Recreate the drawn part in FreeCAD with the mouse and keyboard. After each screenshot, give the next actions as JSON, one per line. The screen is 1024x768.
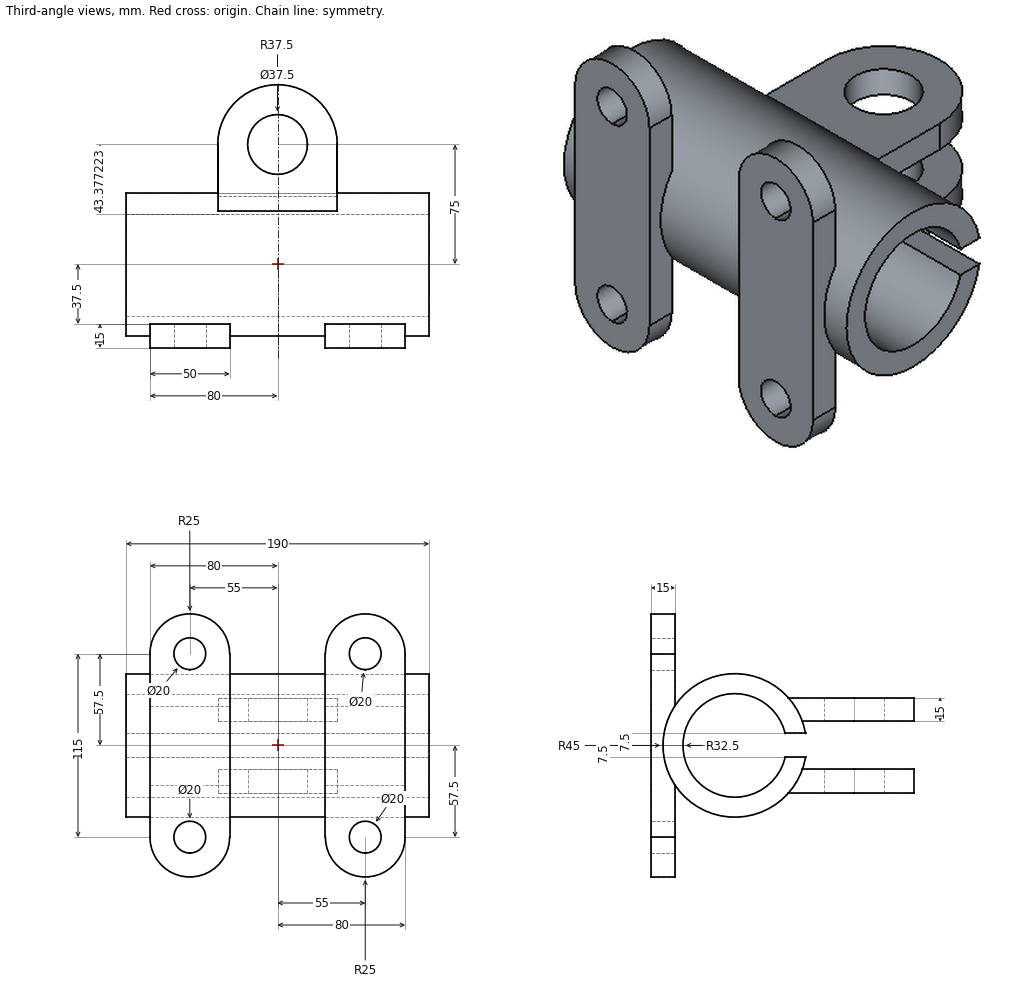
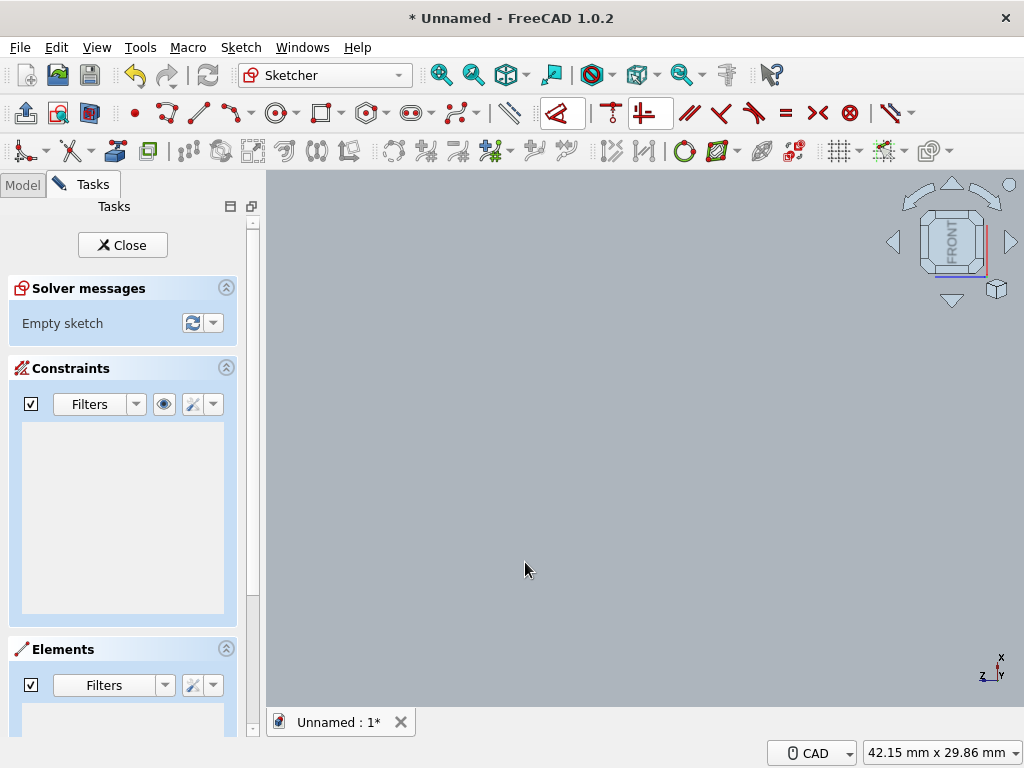
{"action": "left_click", "coordinate": [276, 114]}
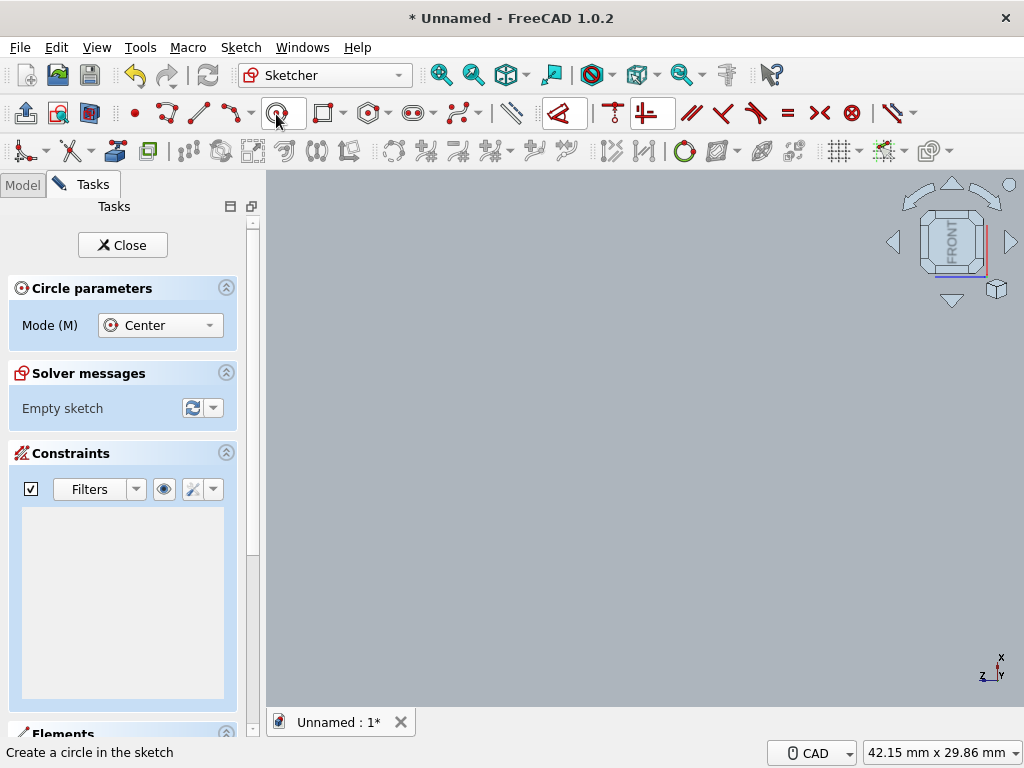
{"action": "left_click", "coordinate": [571, 431]}
{"action": "left_click", "coordinate": [698, 304]}
{"action": "key", "text": "Escape"}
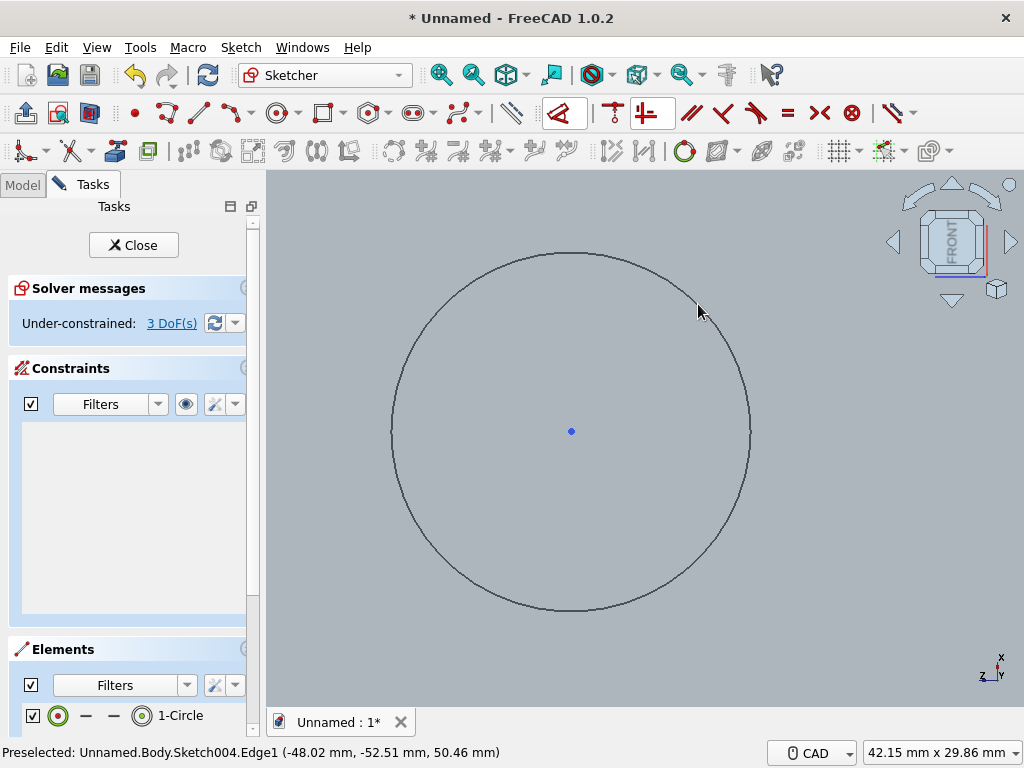
{"action": "left_click", "coordinate": [698, 305]}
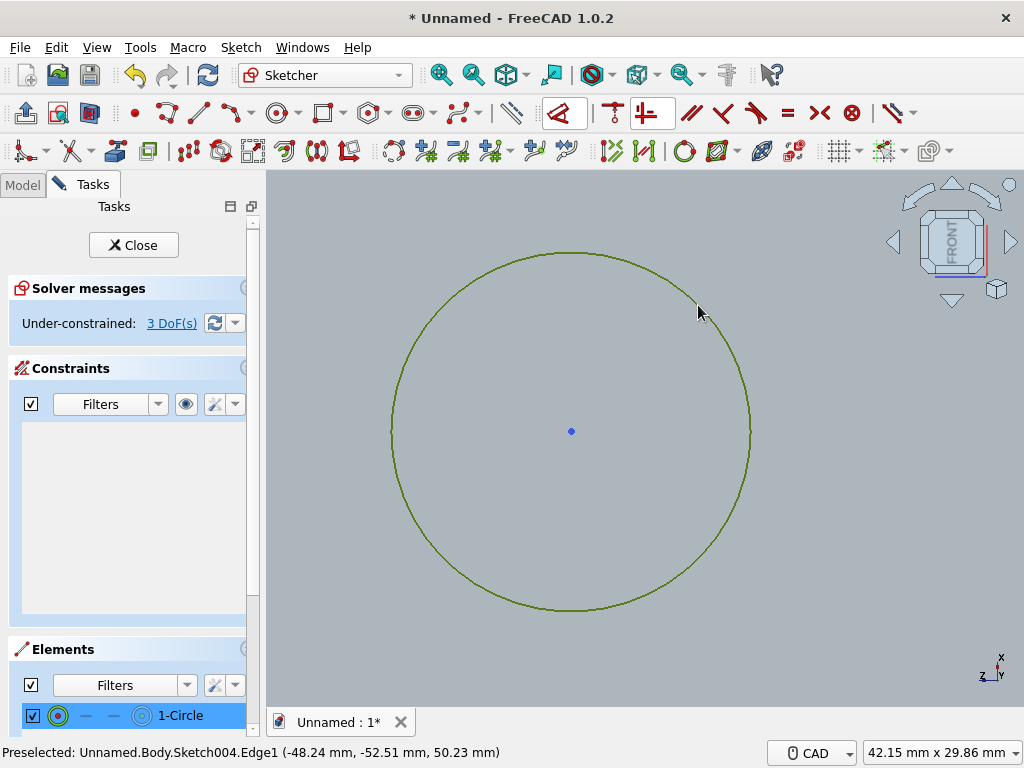
{"action": "left_click", "coordinate": [582, 114]}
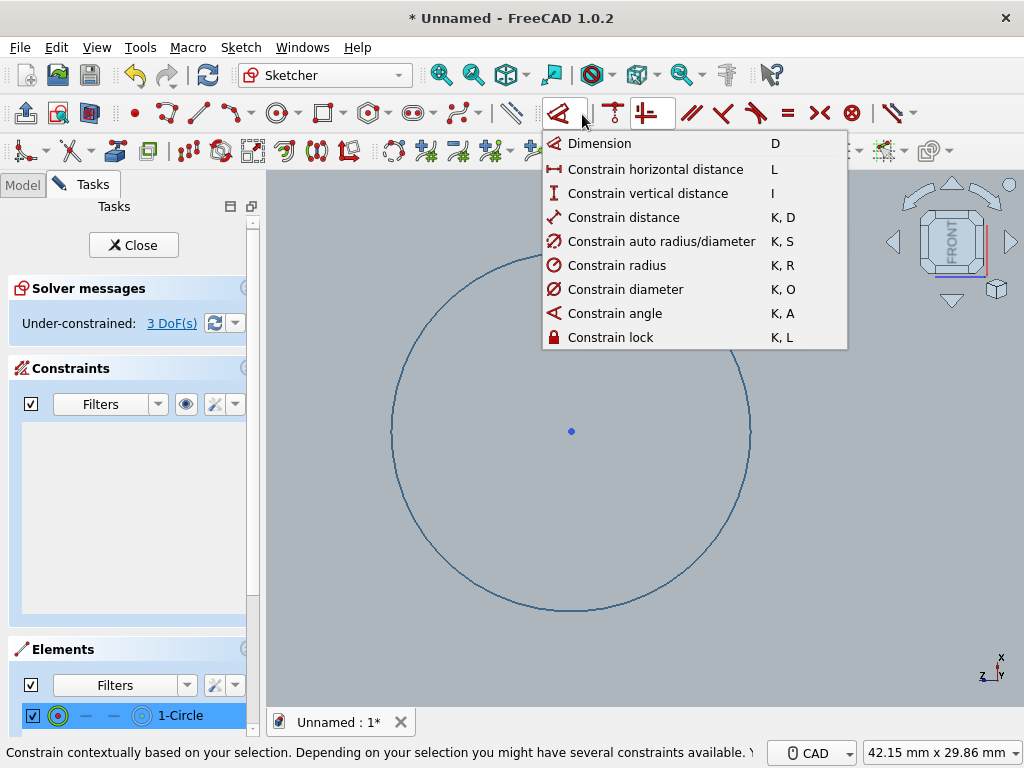
{"action": "left_click", "coordinate": [695, 289]}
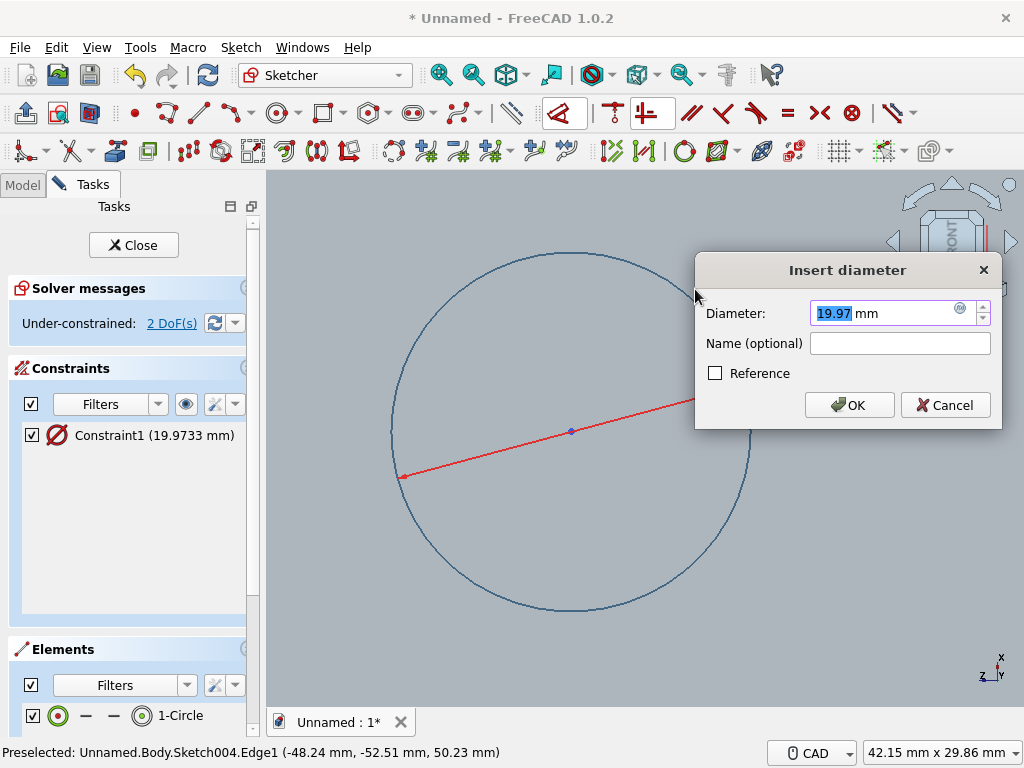
{"action": "type", "text": "20"}
{"action": "key", "text": "Return"}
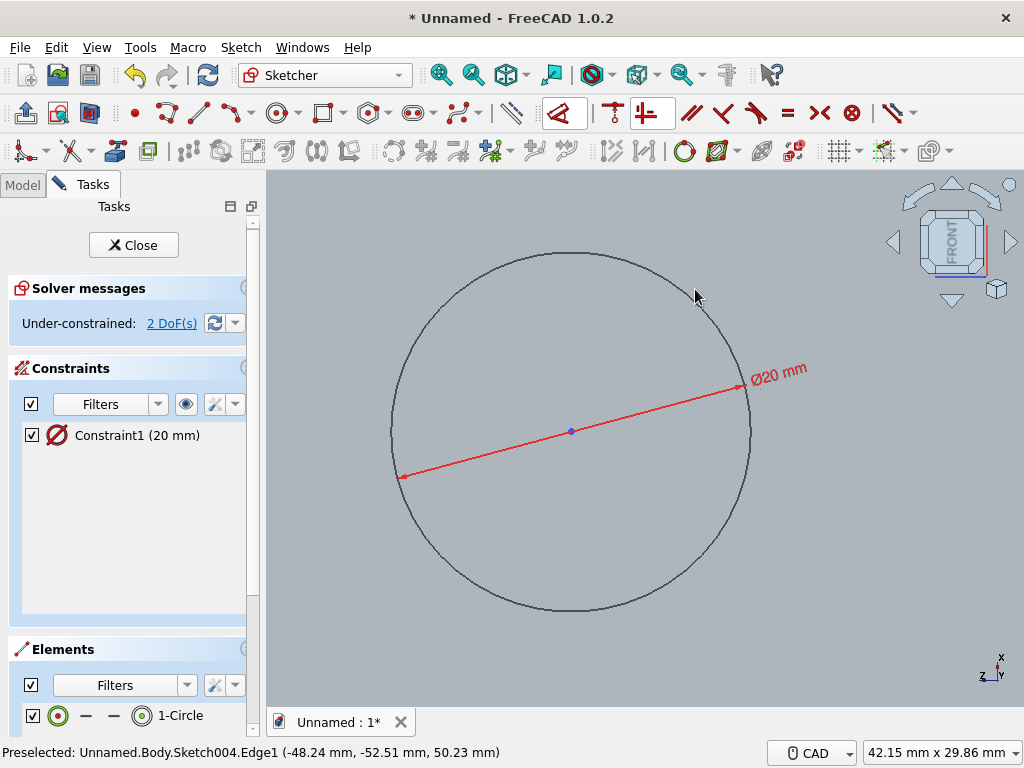
{"action": "left_click", "coordinate": [571, 432]}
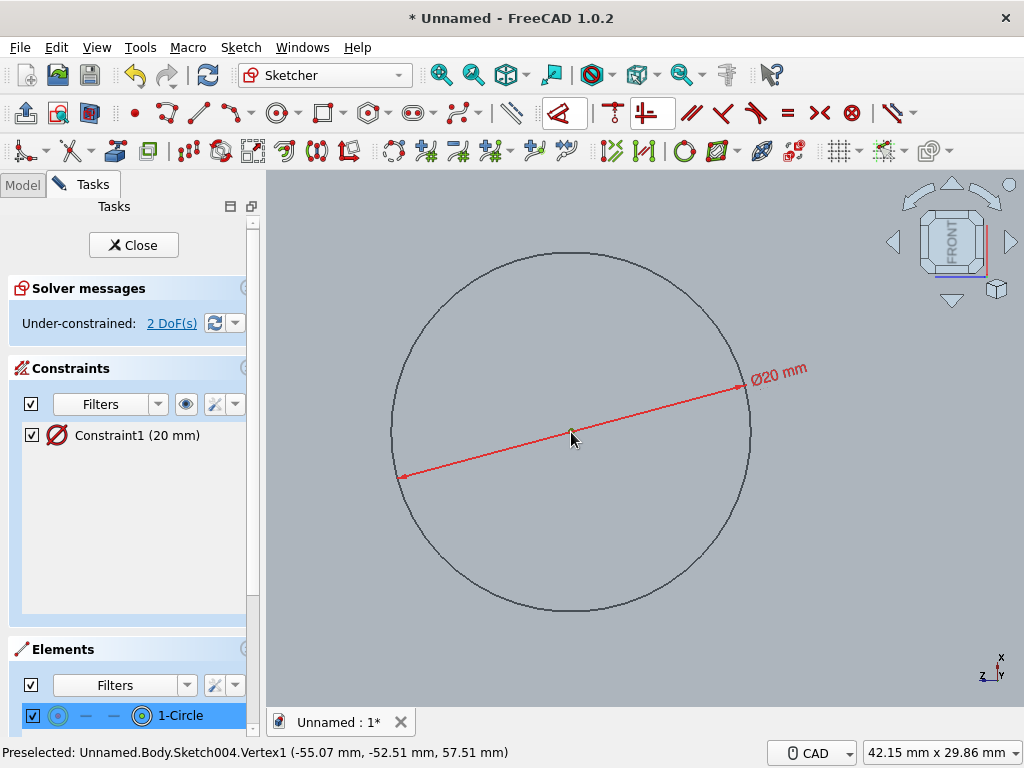
{"action": "left_click", "coordinate": [582, 114]}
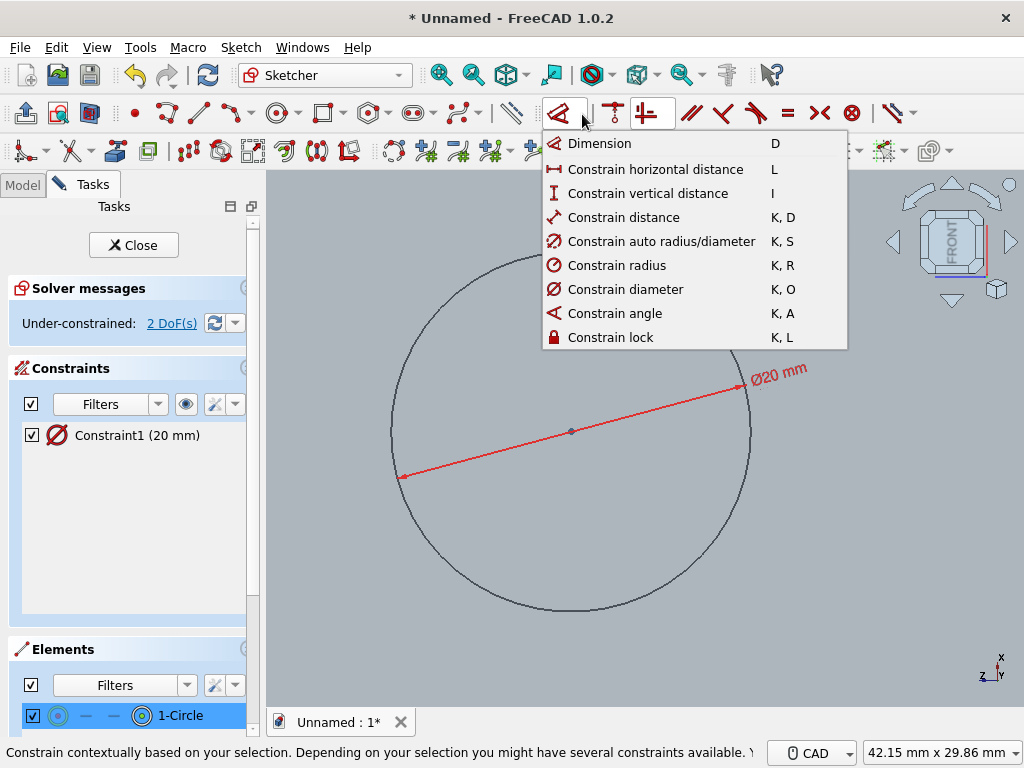
{"action": "left_click", "coordinate": [695, 193]}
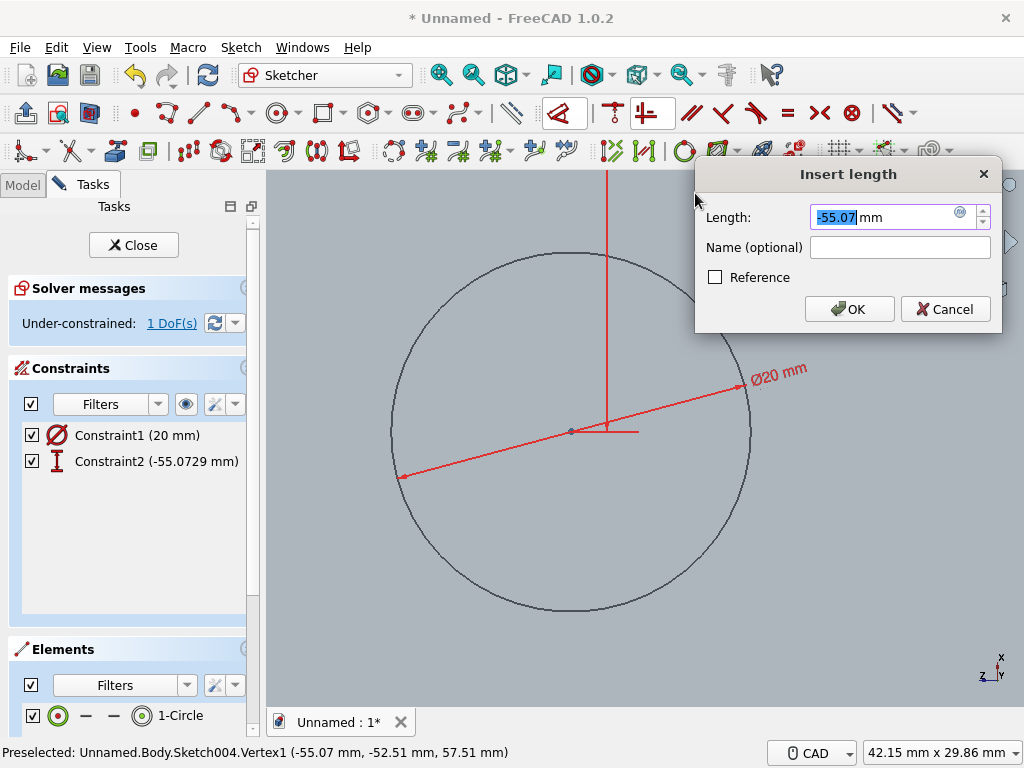
{"action": "type", "text": "-55"}
{"action": "key", "text": "Return"}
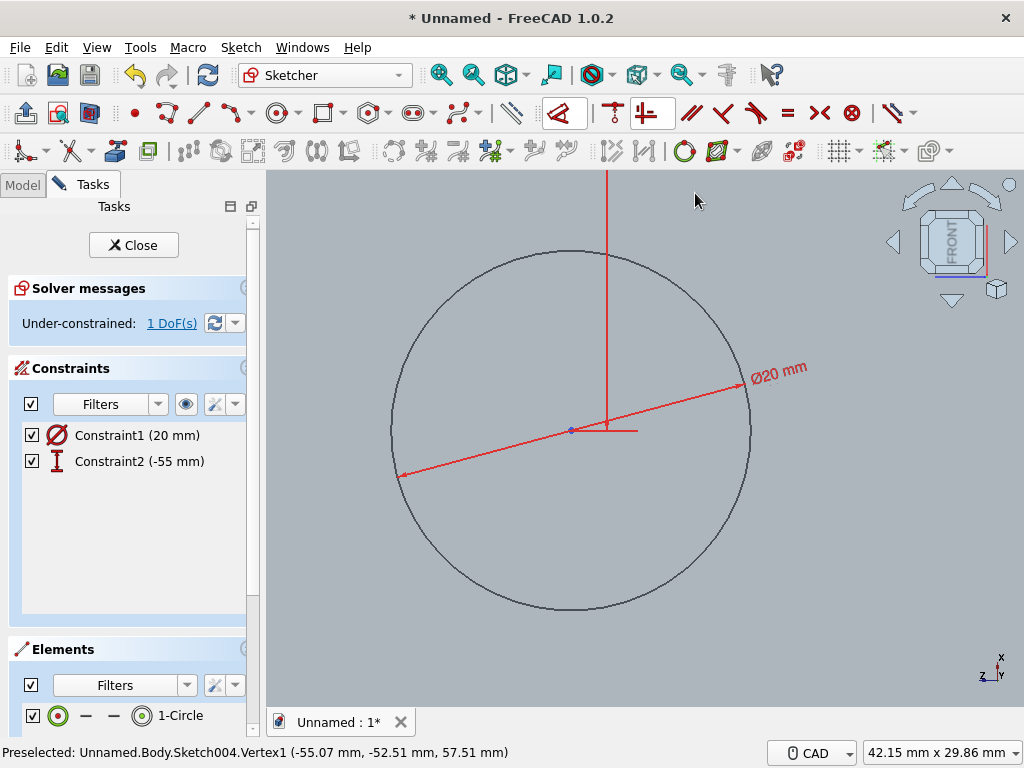
{"action": "left_click", "coordinate": [571, 431]}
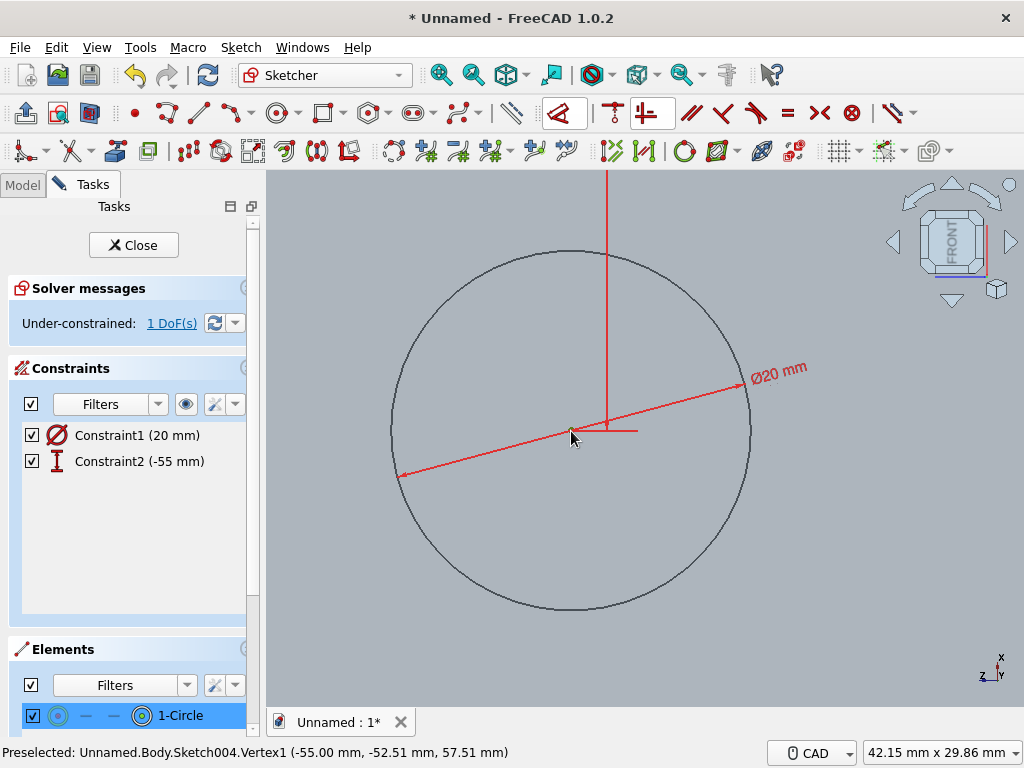
{"action": "left_click", "coordinate": [582, 114]}